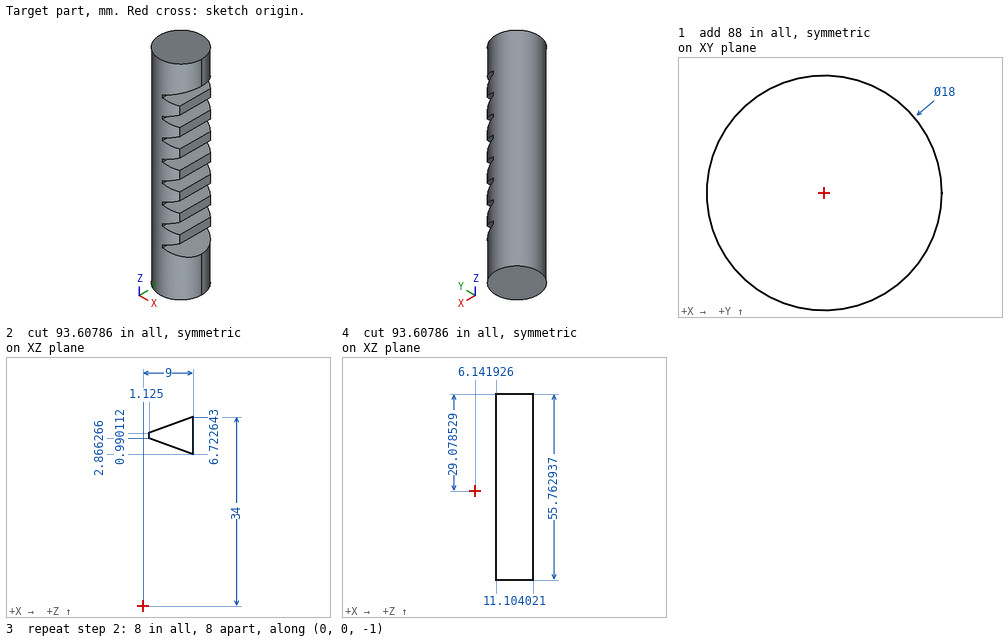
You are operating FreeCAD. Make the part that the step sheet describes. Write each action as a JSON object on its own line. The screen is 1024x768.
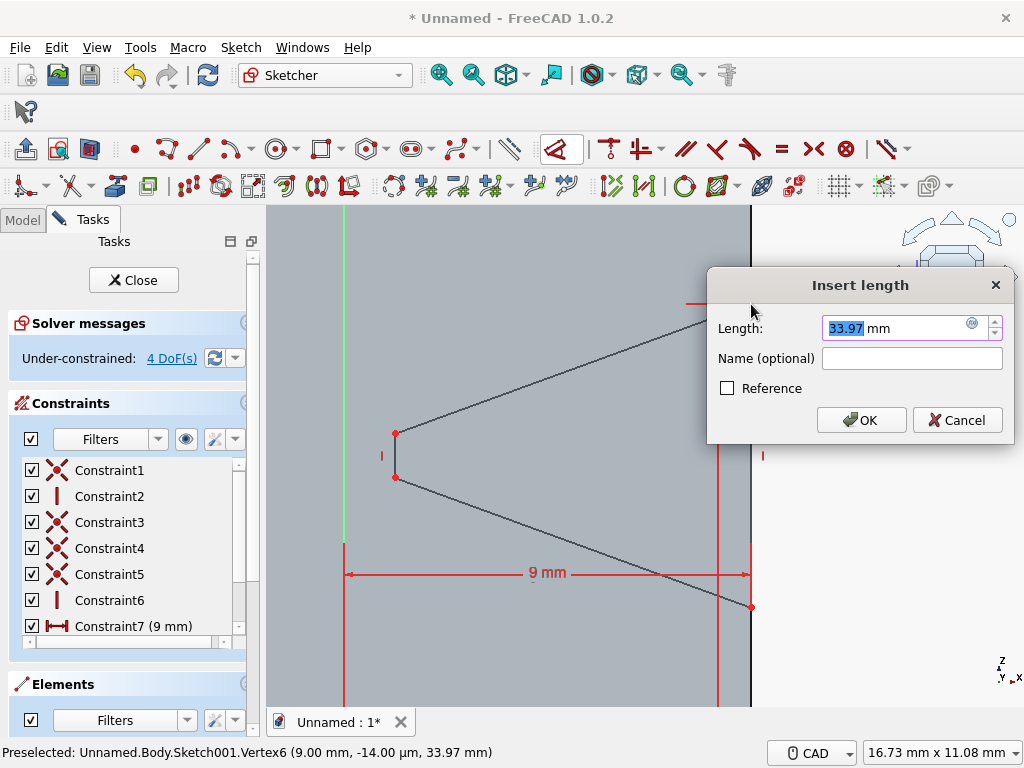
{"action": "type", "text": "34"}
{"action": "key", "text": "Return"}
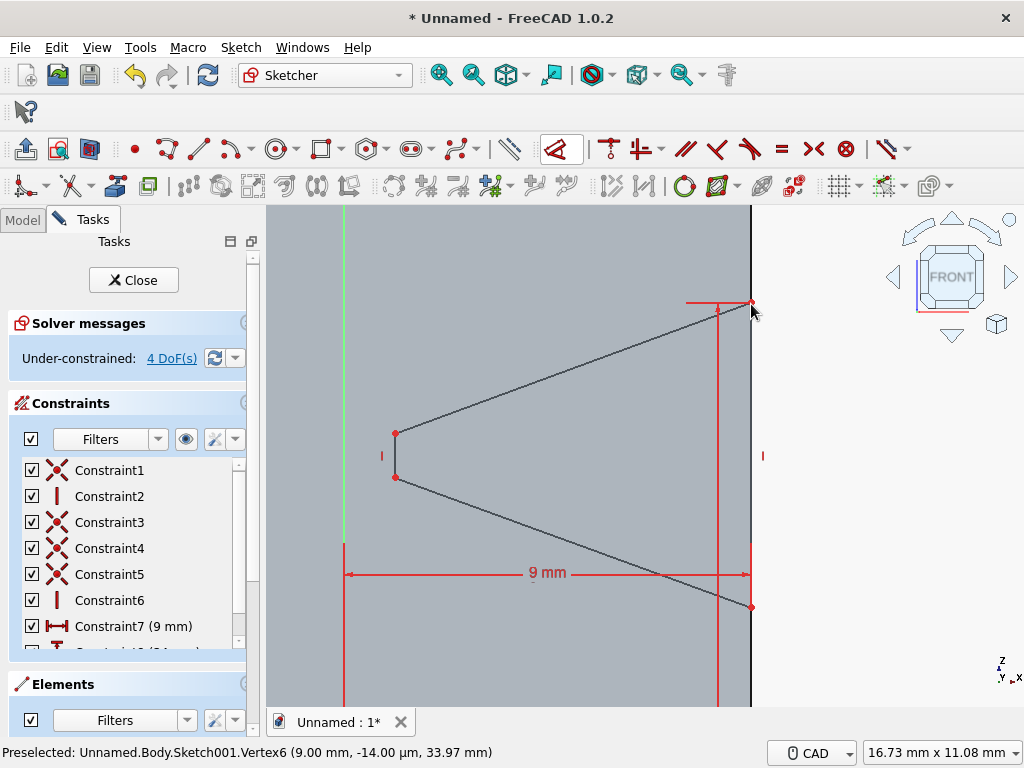
{"action": "left_click", "coordinate": [395, 478]}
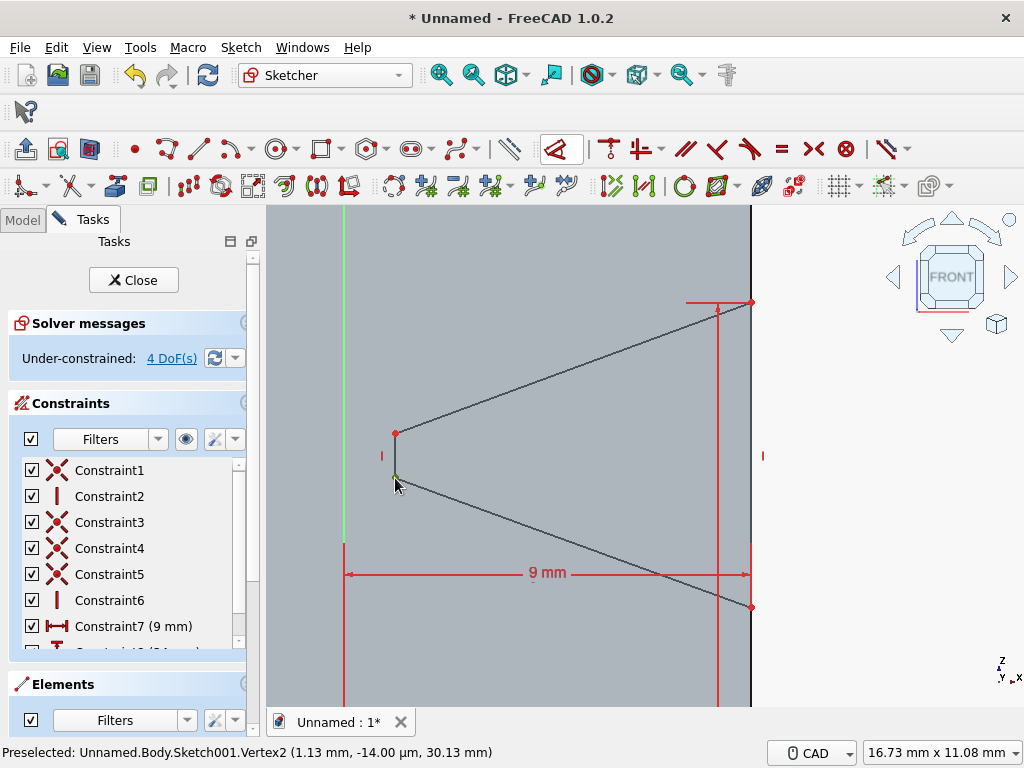
{"action": "left_click", "coordinate": [578, 150]}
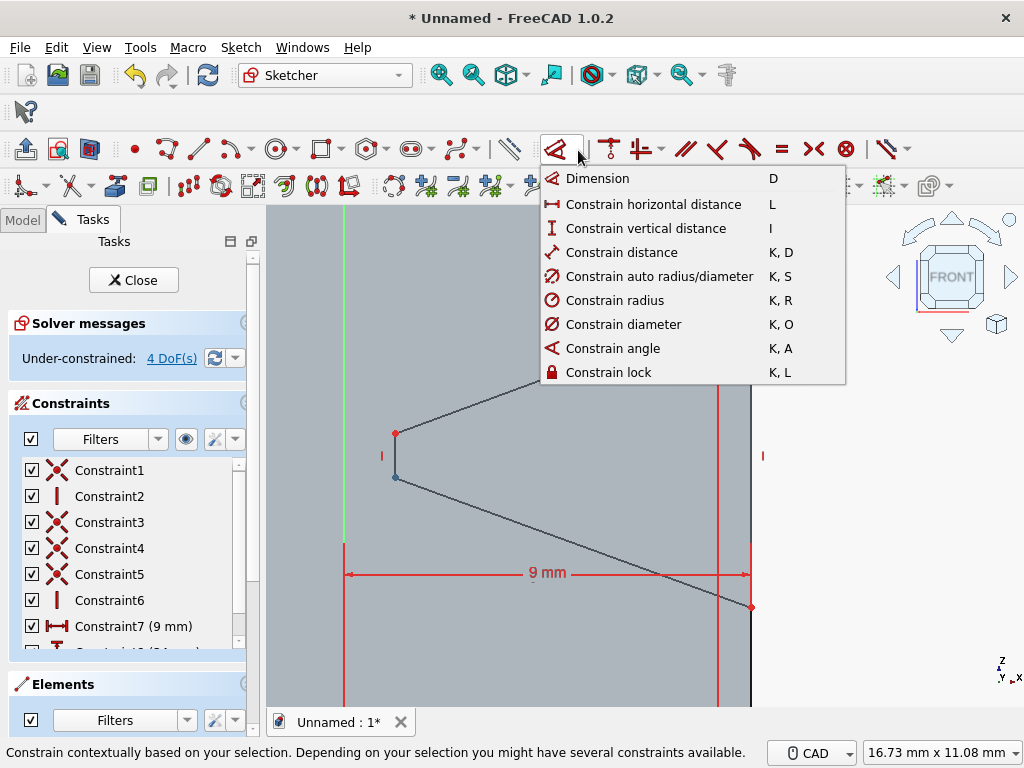
{"action": "left_click", "coordinate": [693, 204]}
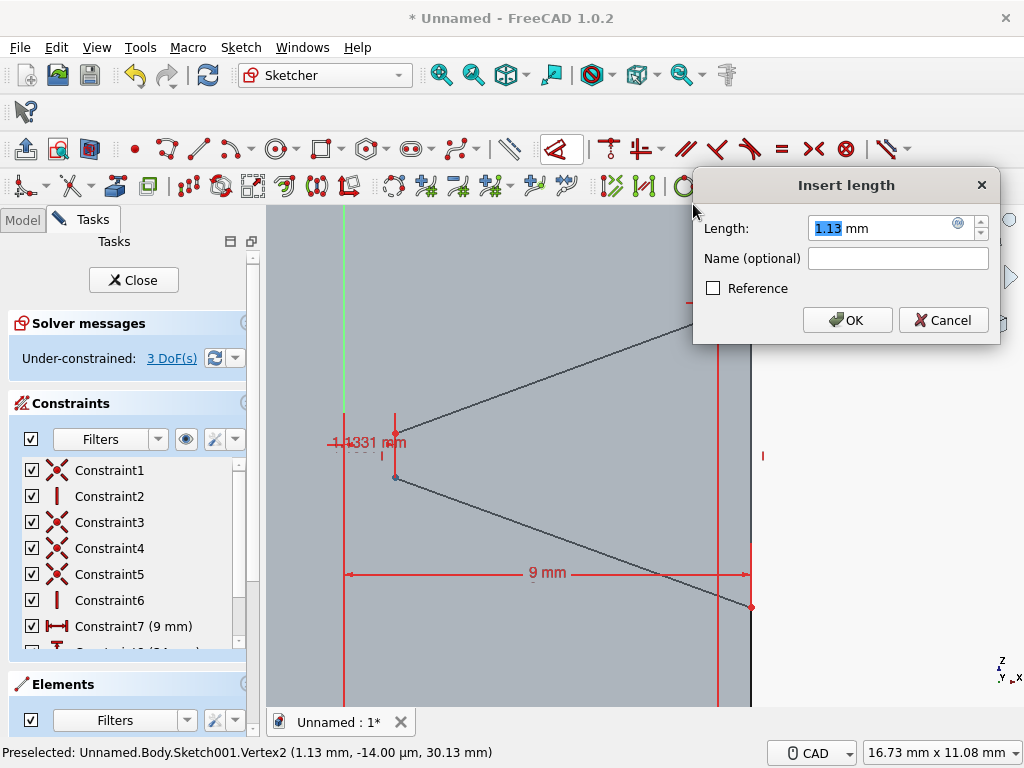
{"action": "type", "text": "1.125"}
{"action": "key", "text": "Return"}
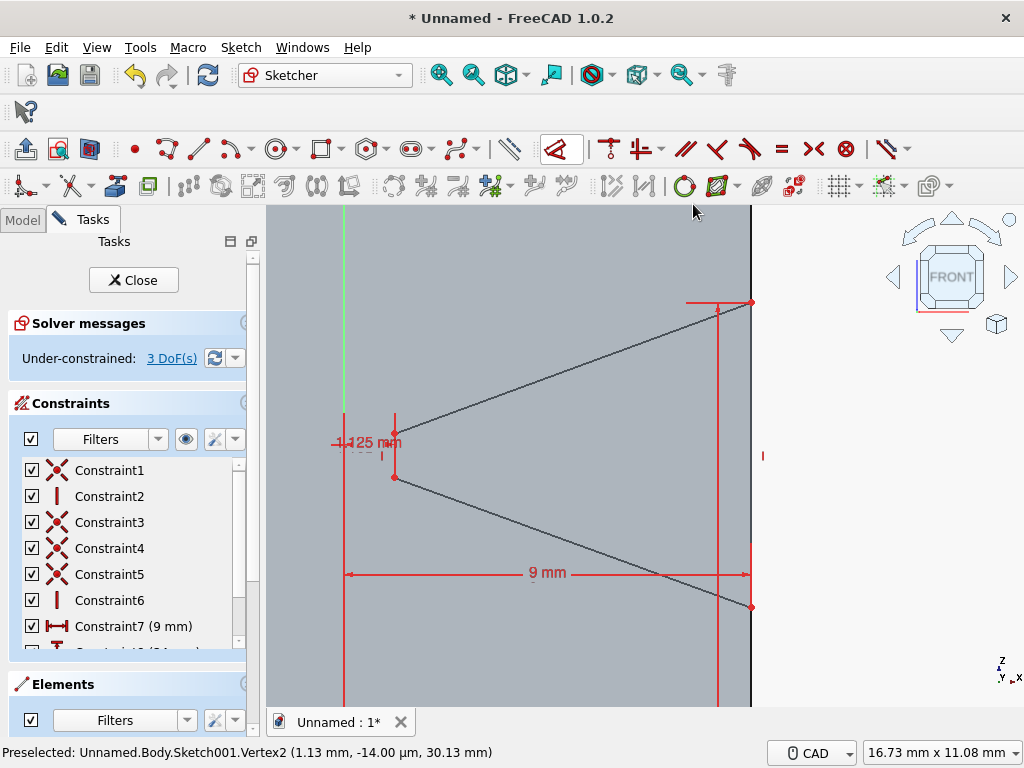
{"action": "left_click", "coordinate": [395, 465]}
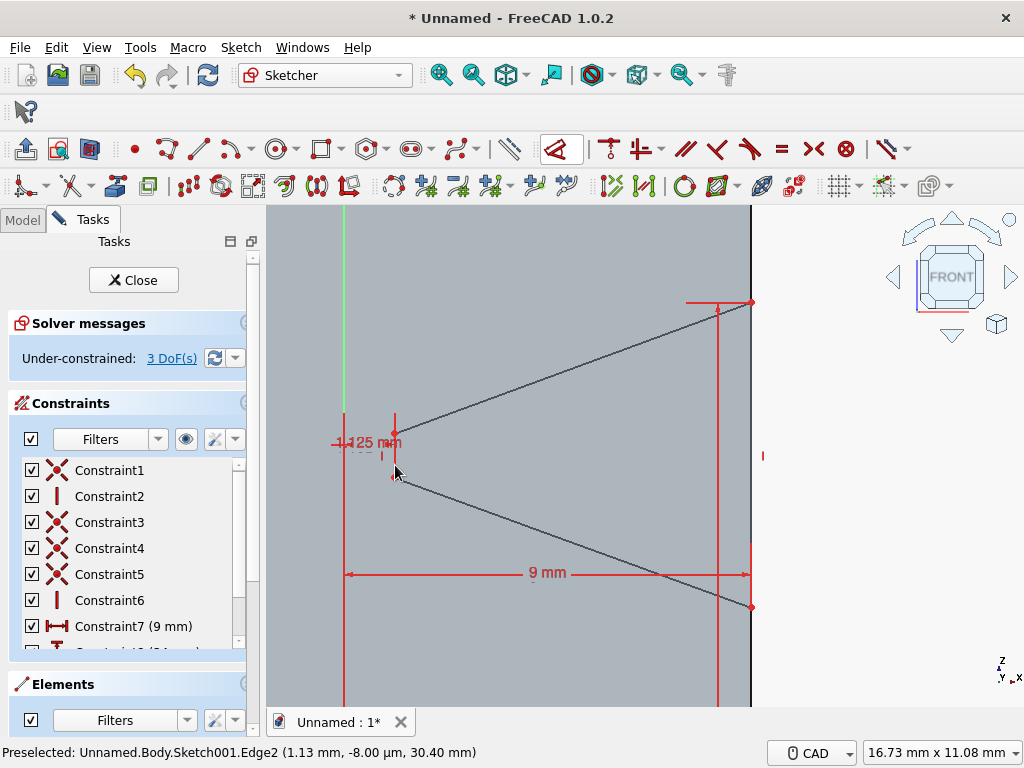
{"action": "key", "text": "i"}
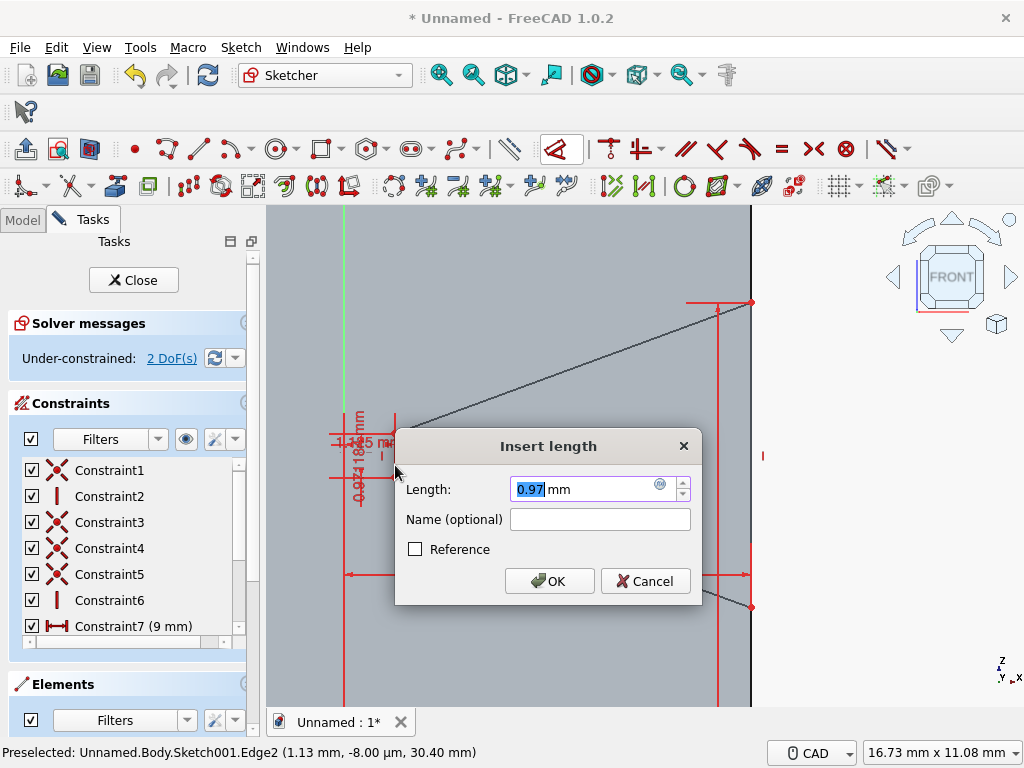
{"action": "type", "text": "0.990112"}
{"action": "key", "text": "Return"}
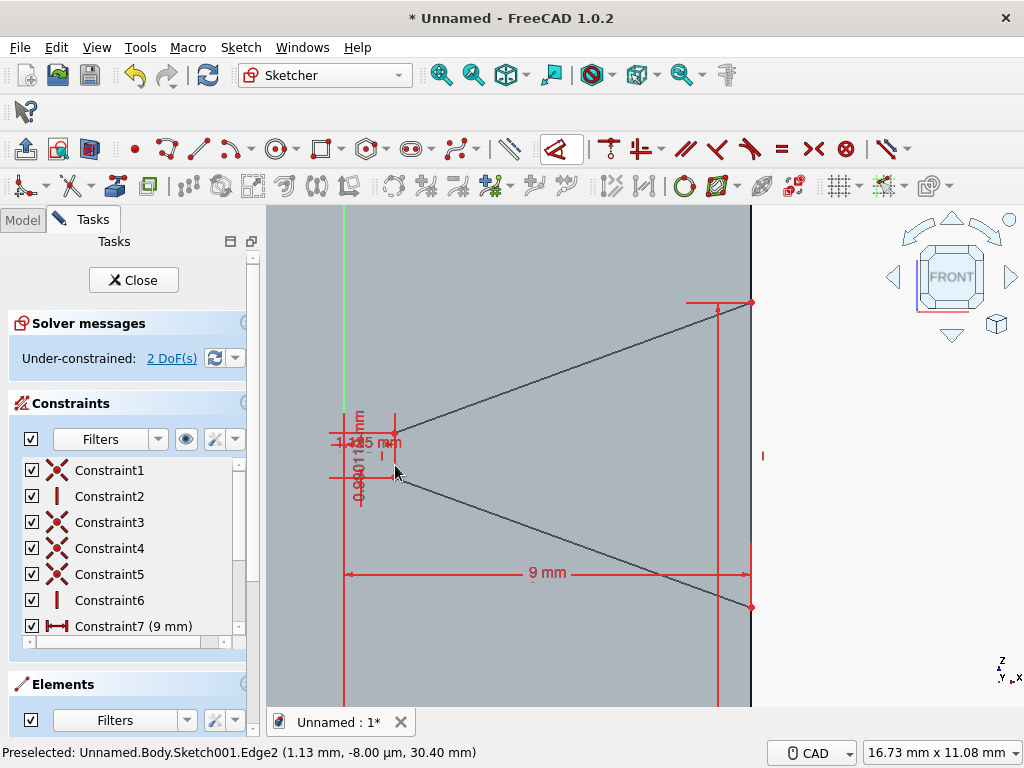
{"action": "left_click", "coordinate": [751, 394]}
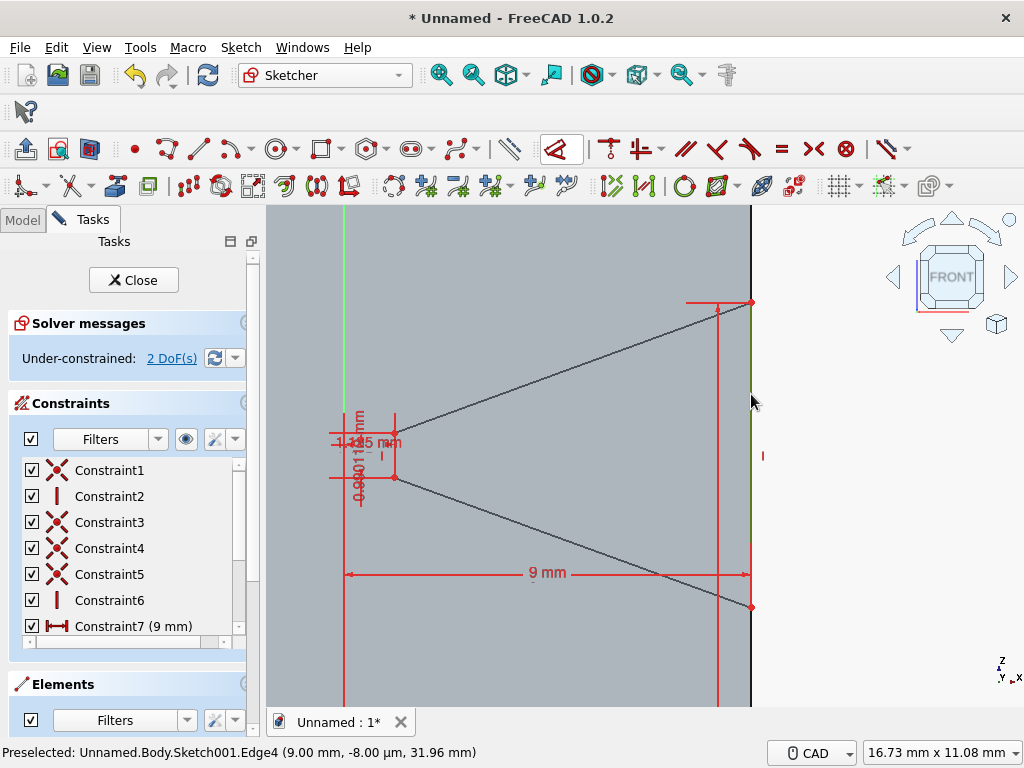
{"action": "left_click", "coordinate": [578, 150]}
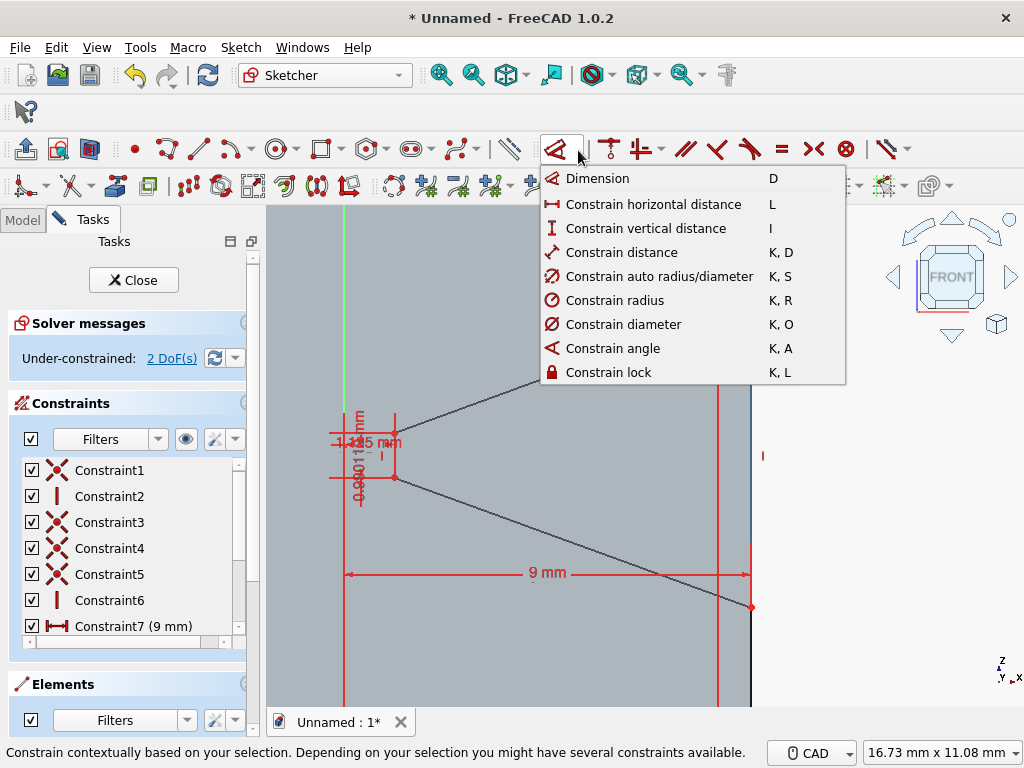
{"action": "left_click", "coordinate": [693, 228]}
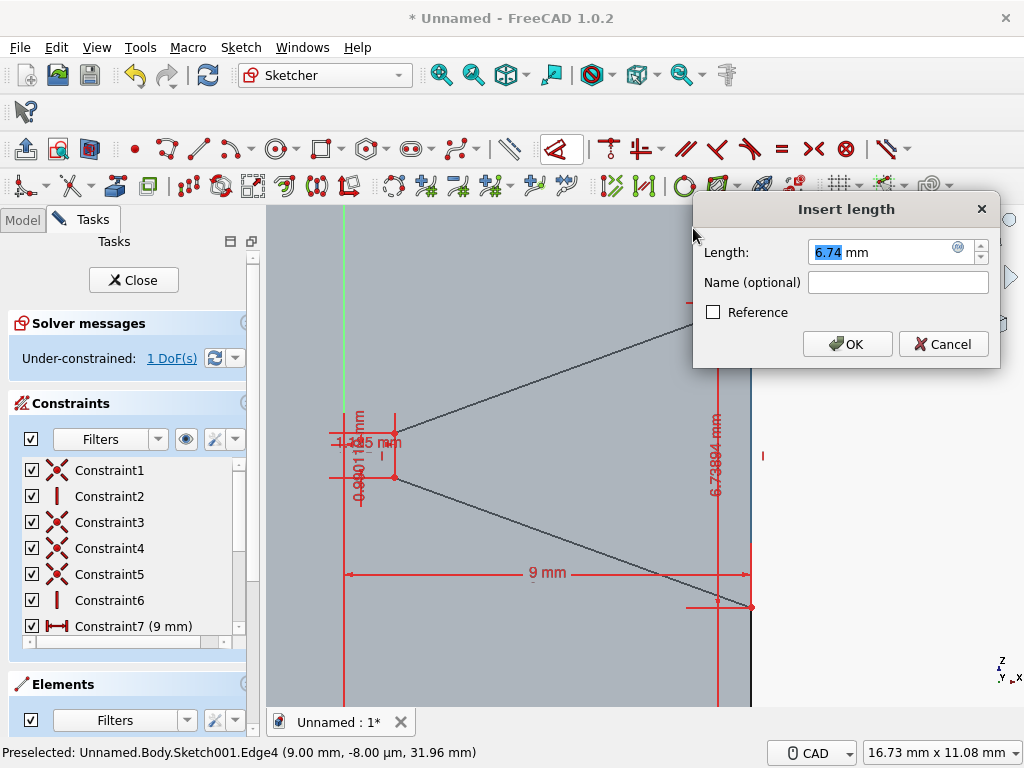
{"action": "type", "text": "6.722643"}
{"action": "key", "text": "Return"}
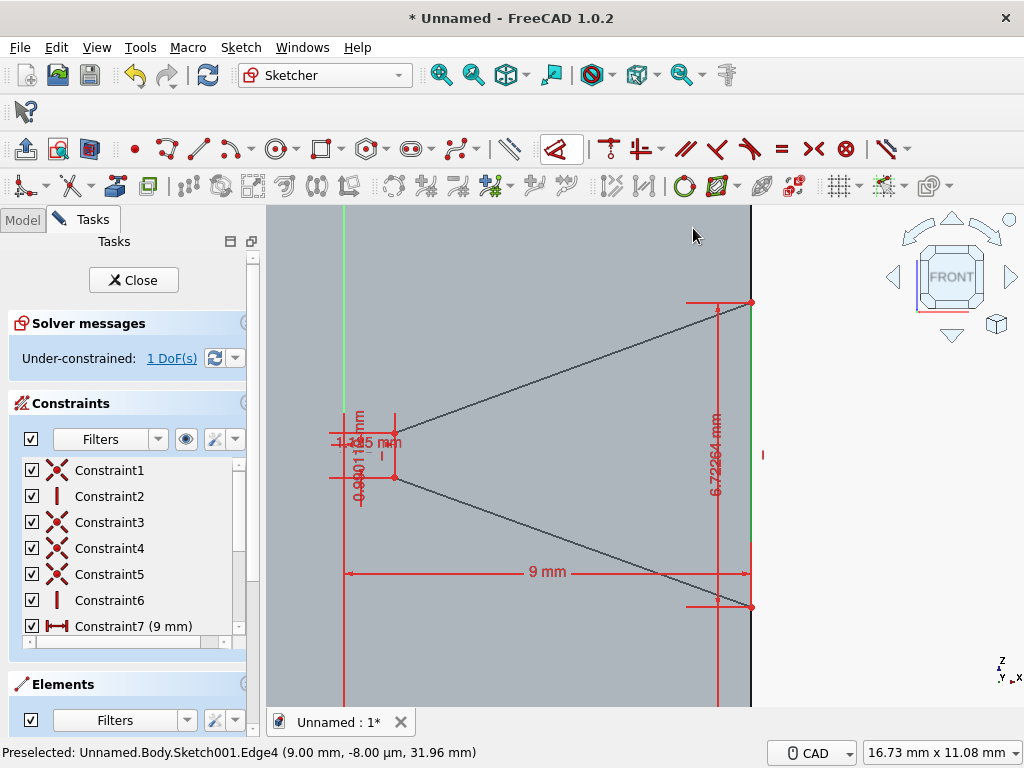
{"action": "left_click", "coordinate": [644, 568]}